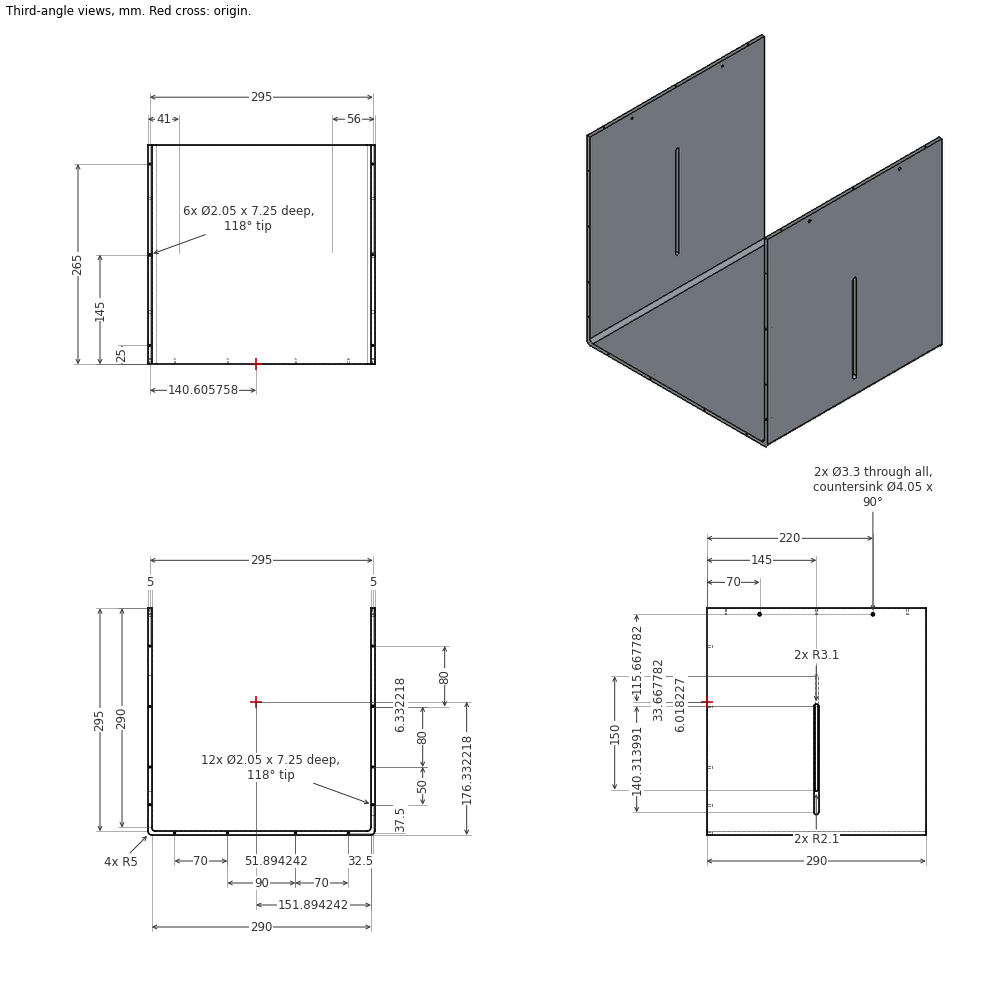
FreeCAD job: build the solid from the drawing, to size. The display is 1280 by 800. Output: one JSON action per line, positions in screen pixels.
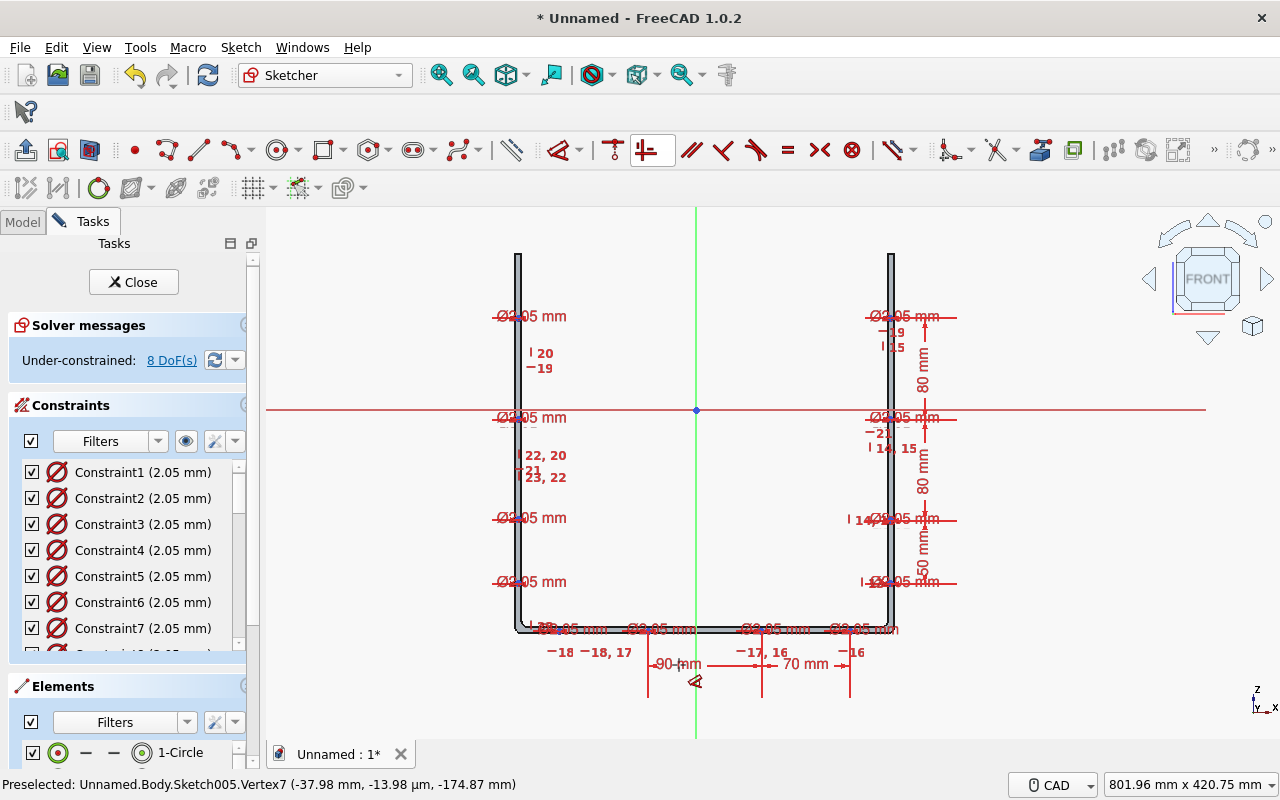
{"action": "left_click", "coordinate": [648, 631]}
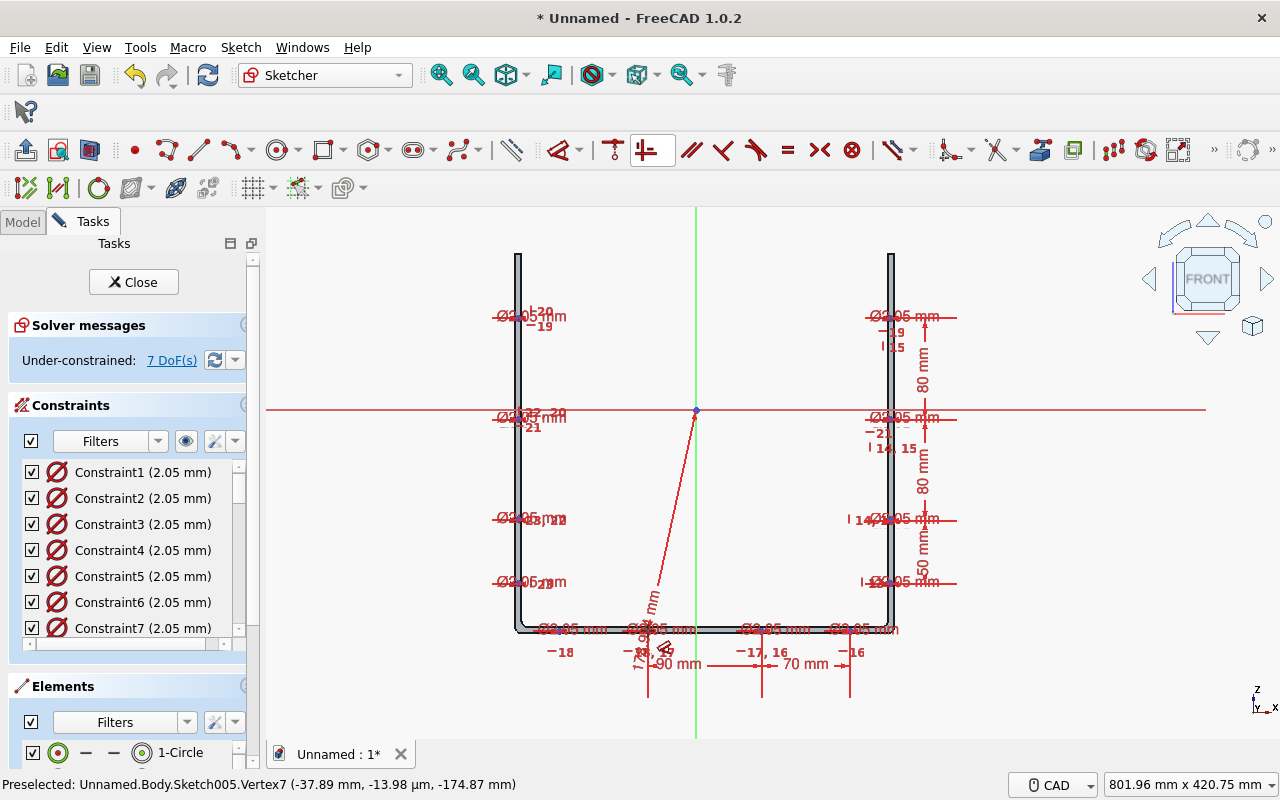
{"action": "left_click", "coordinate": [559, 631]}
{"action": "left_click", "coordinate": [604, 665]}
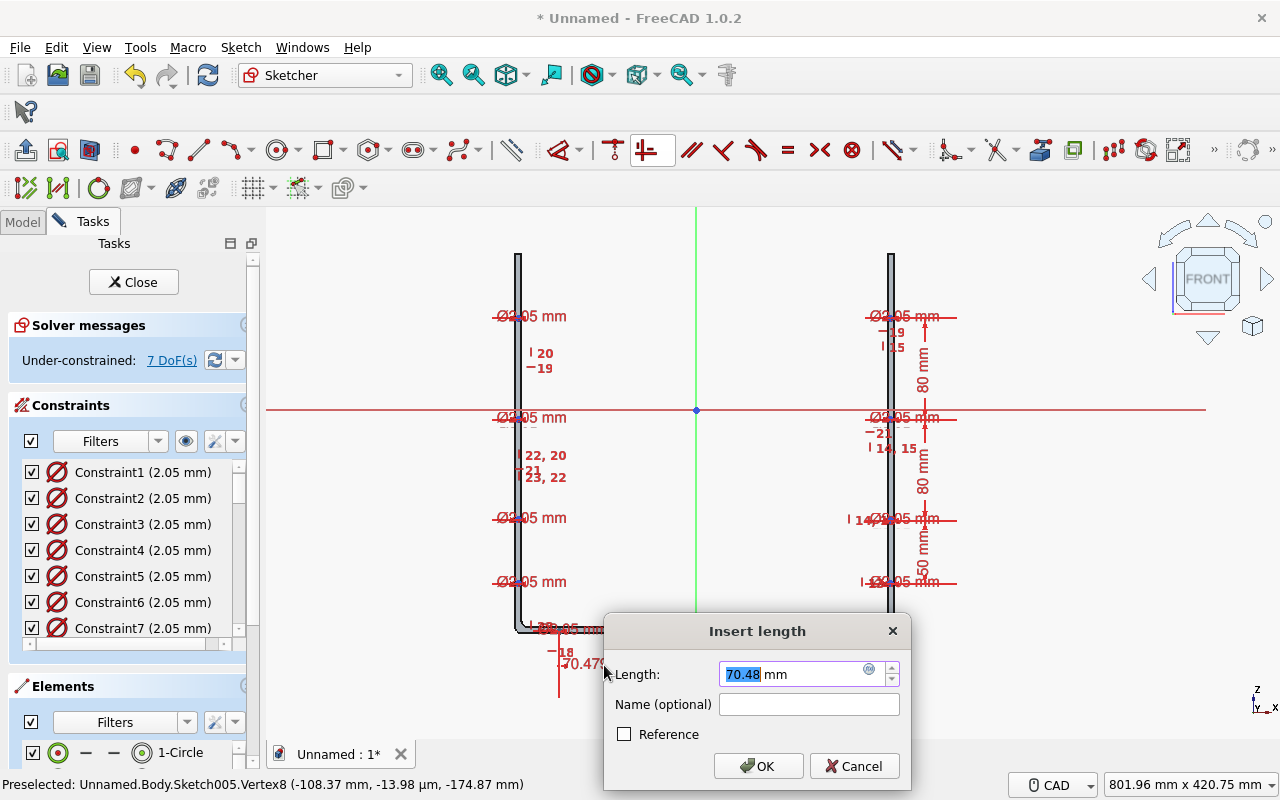
{"action": "type", "text": "70"}
{"action": "key", "text": "Return"}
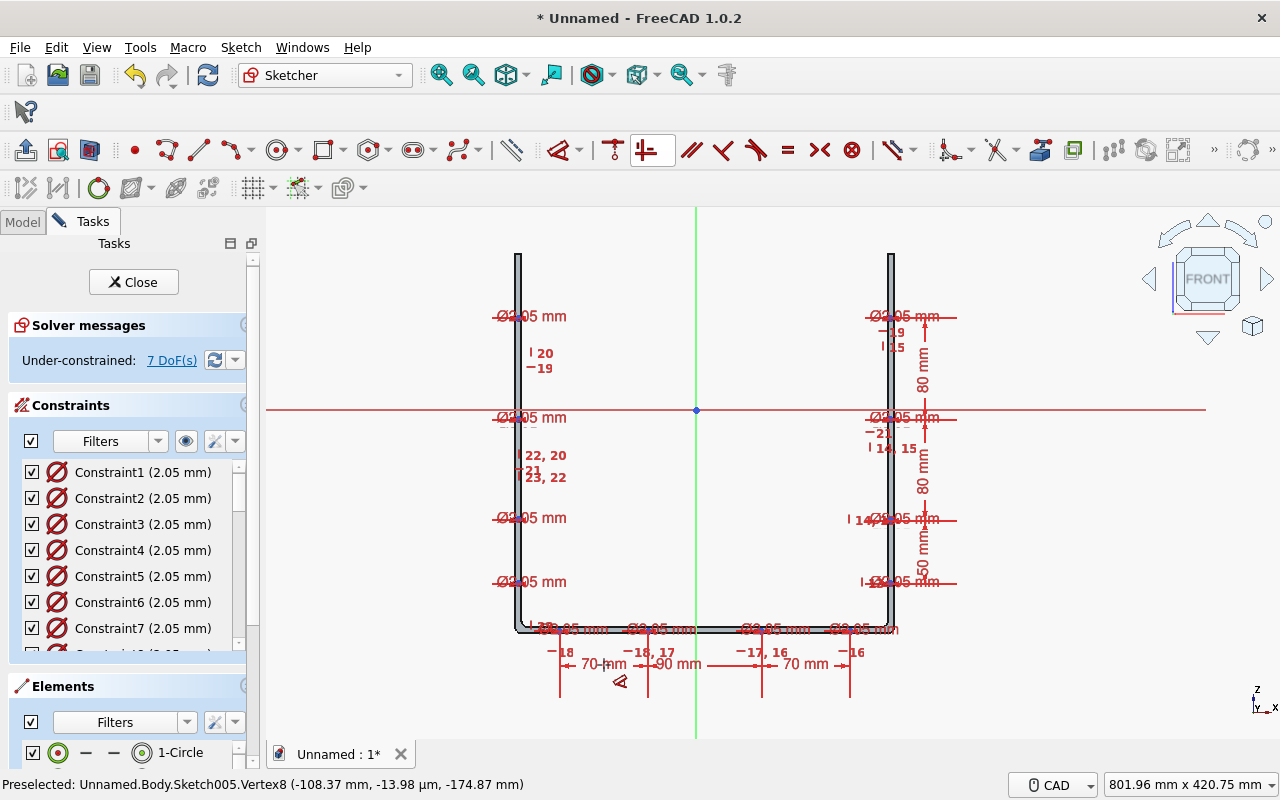
{"action": "left_click", "coordinate": [518, 420]}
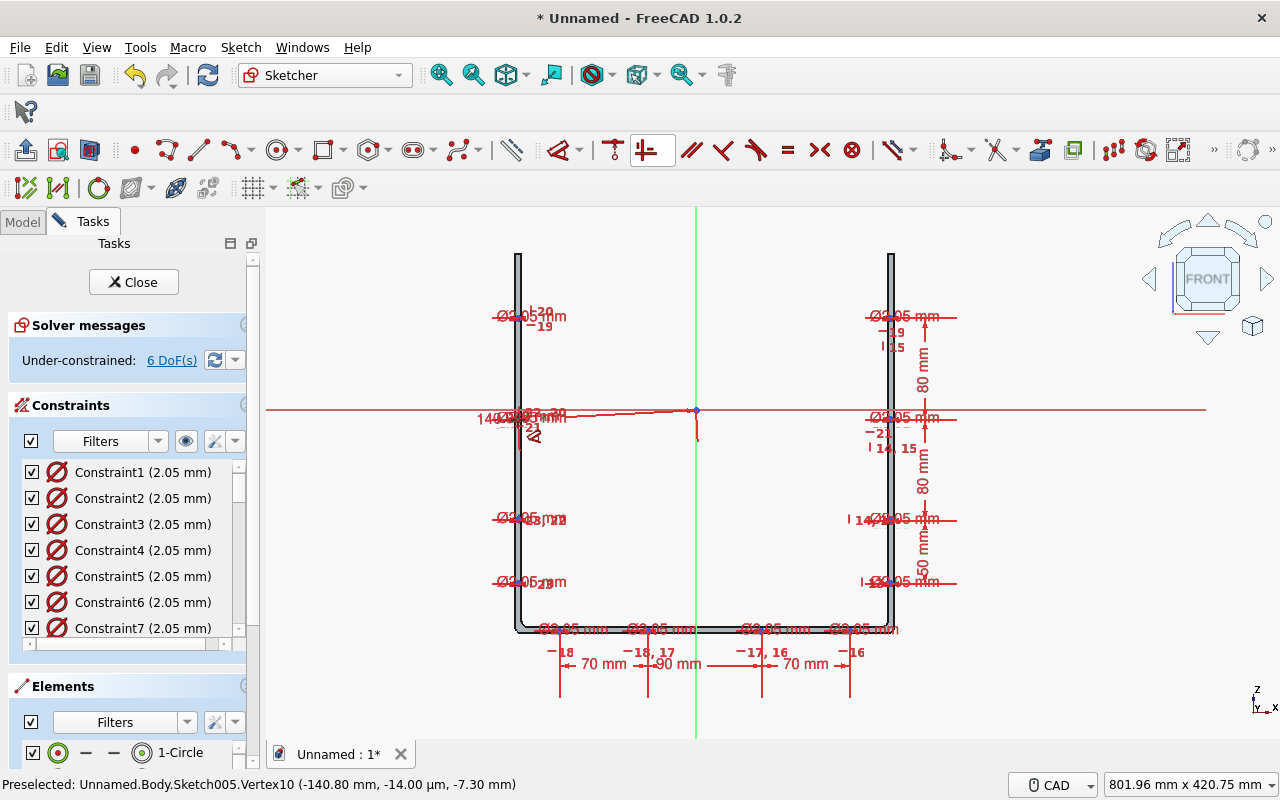
{"action": "left_click", "coordinate": [518, 520]}
{"action": "left_click", "coordinate": [484, 470]}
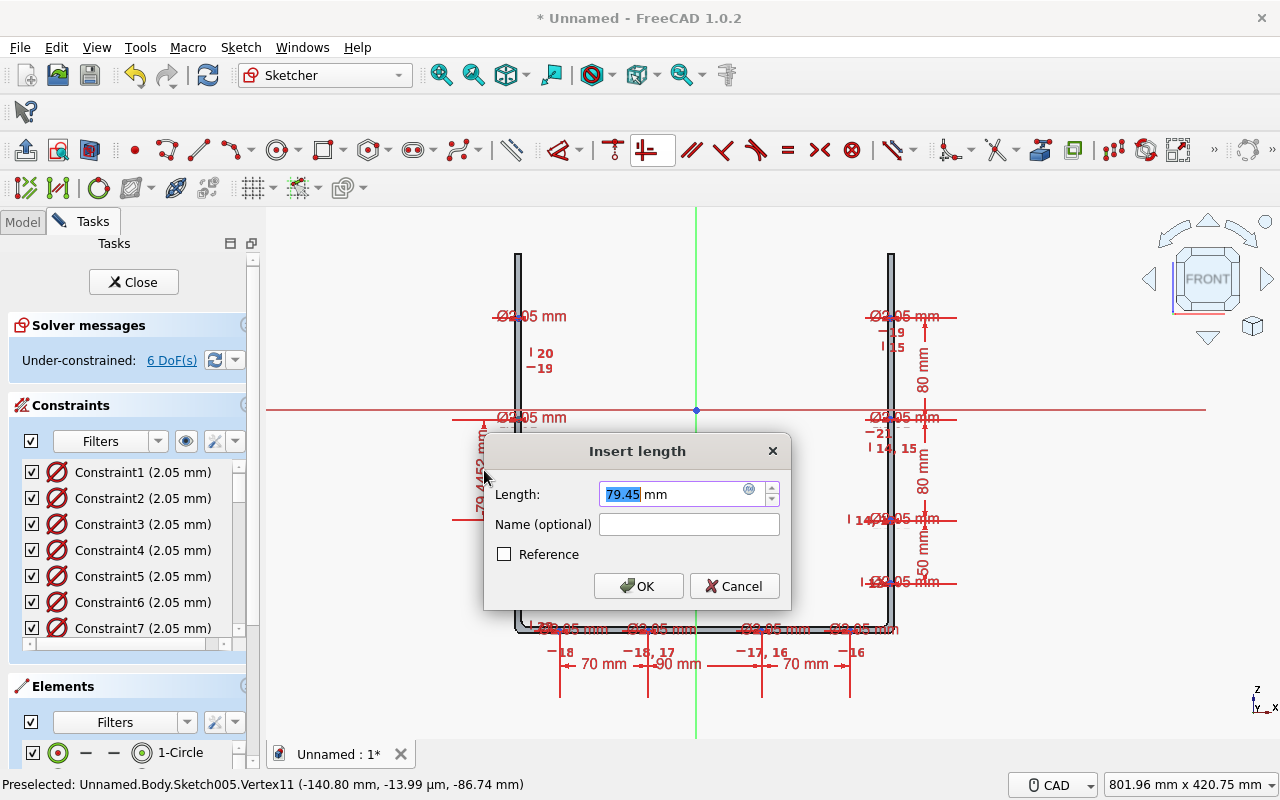
{"action": "type", "text": "80"}
{"action": "key", "text": "Return"}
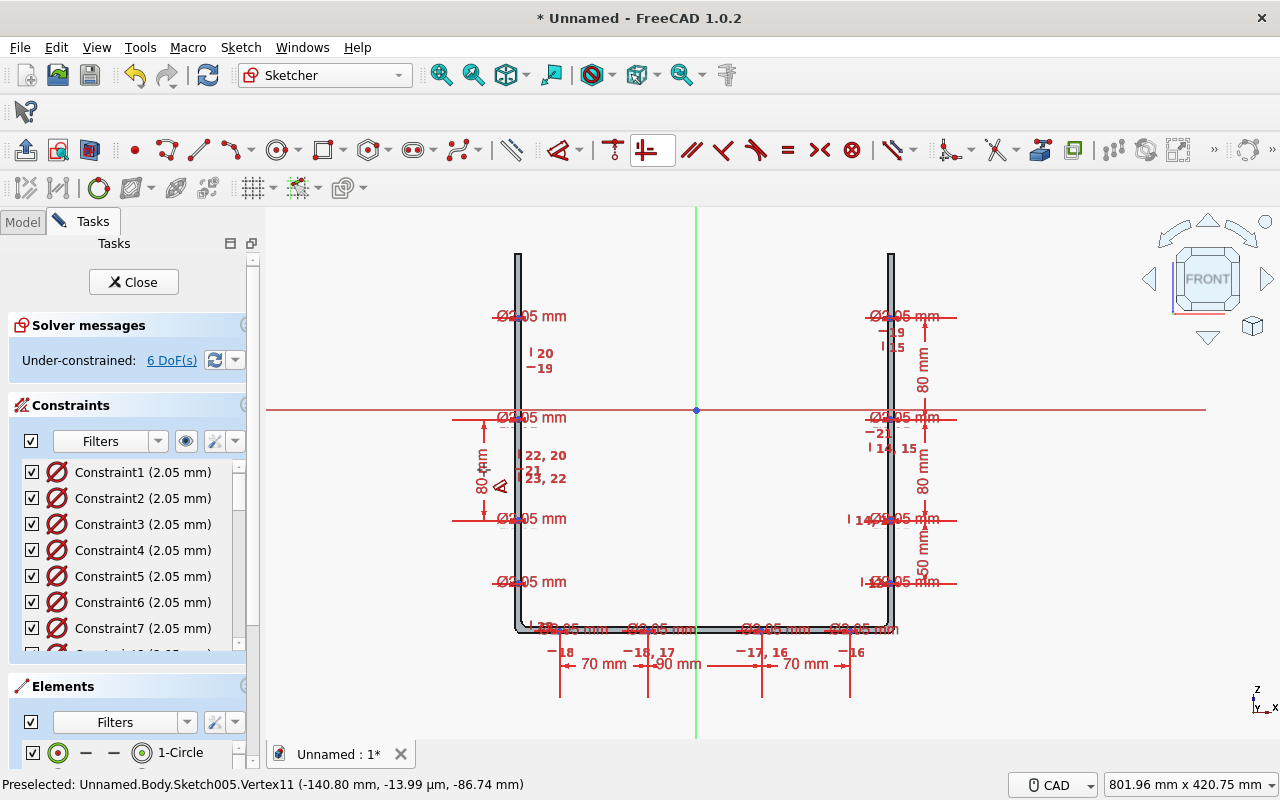
{"action": "left_click", "coordinate": [518, 521]}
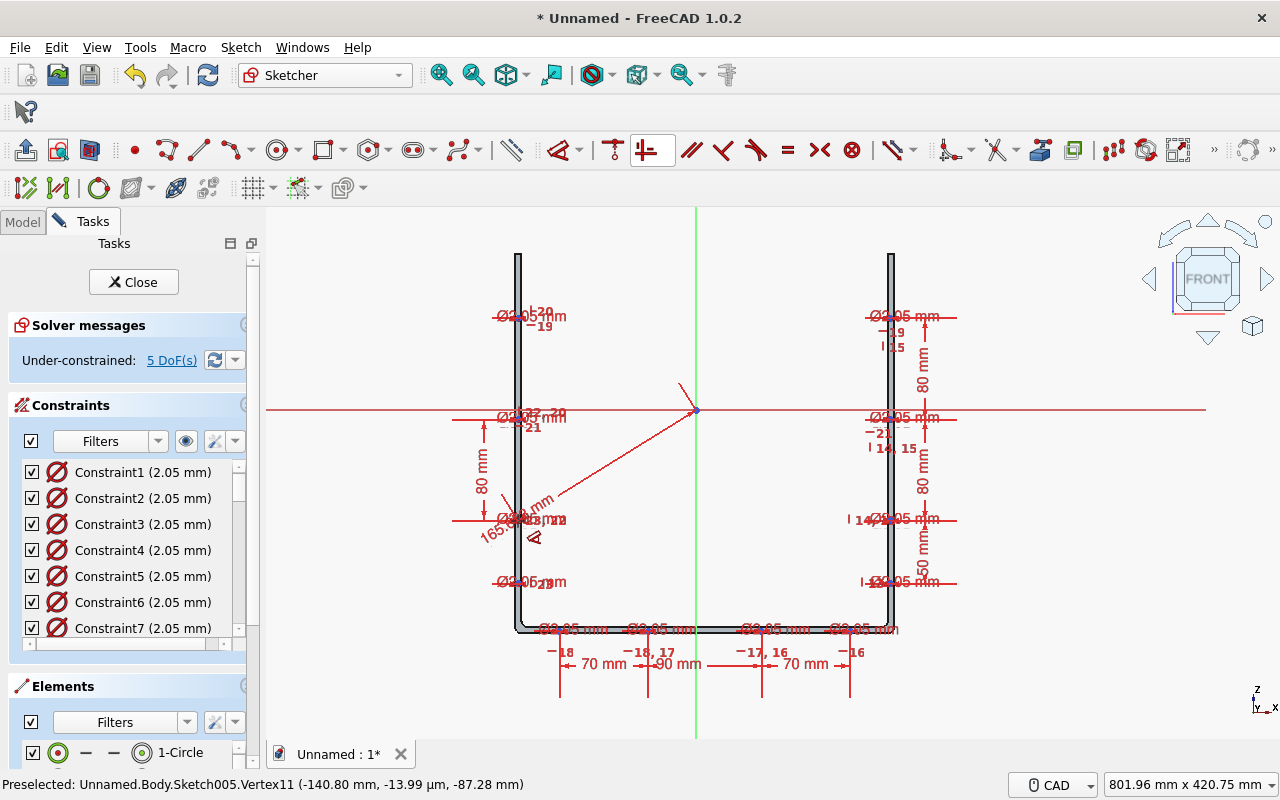
{"action": "left_click", "coordinate": [518, 584]}
{"action": "left_click", "coordinate": [484, 552]}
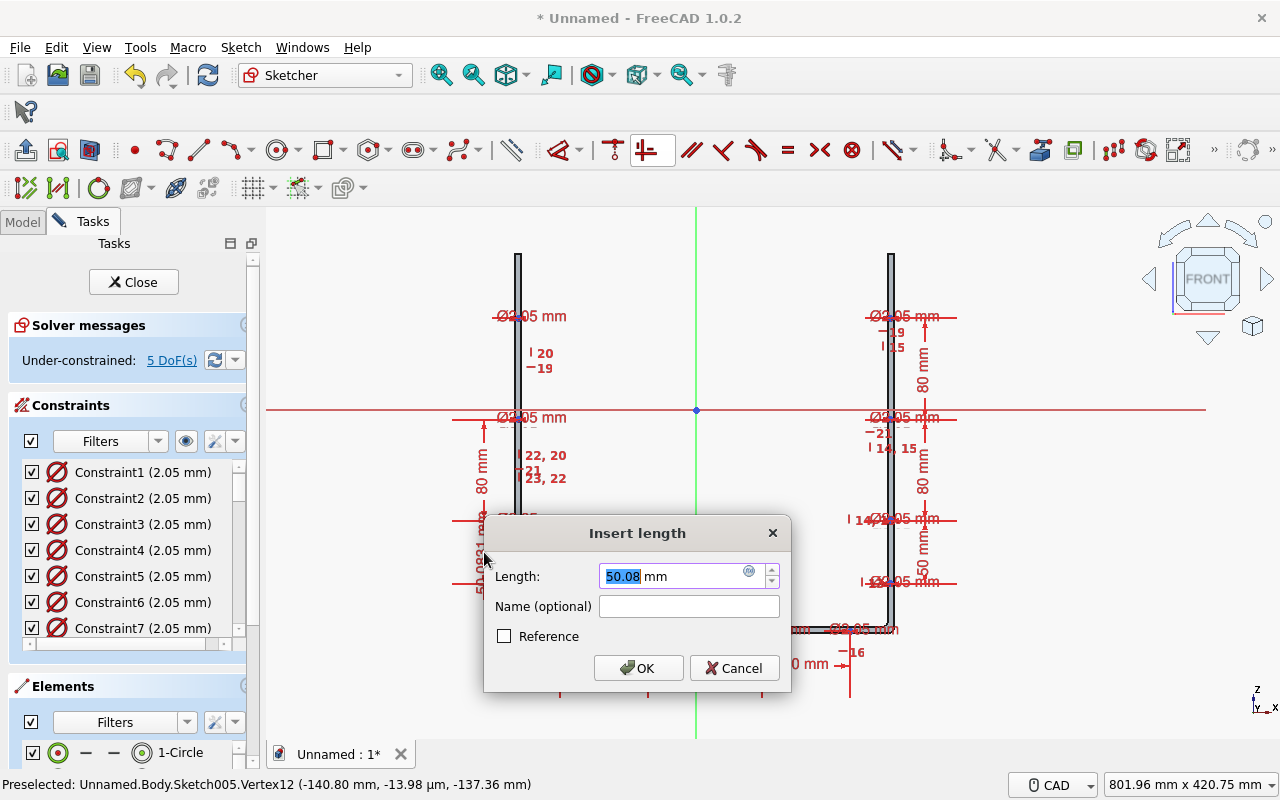
{"action": "type", "text": "50"}
{"action": "key", "text": "Return"}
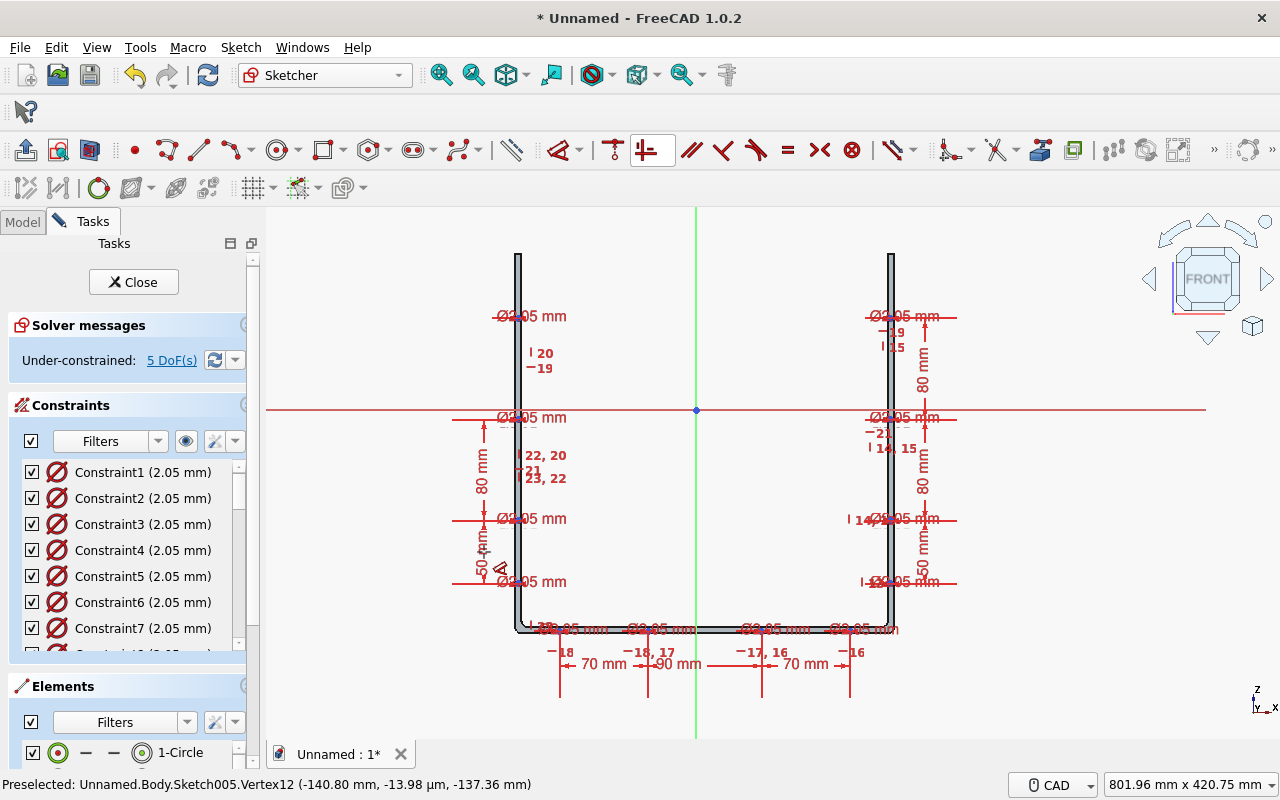
{"action": "left_click", "coordinate": [891, 318]}